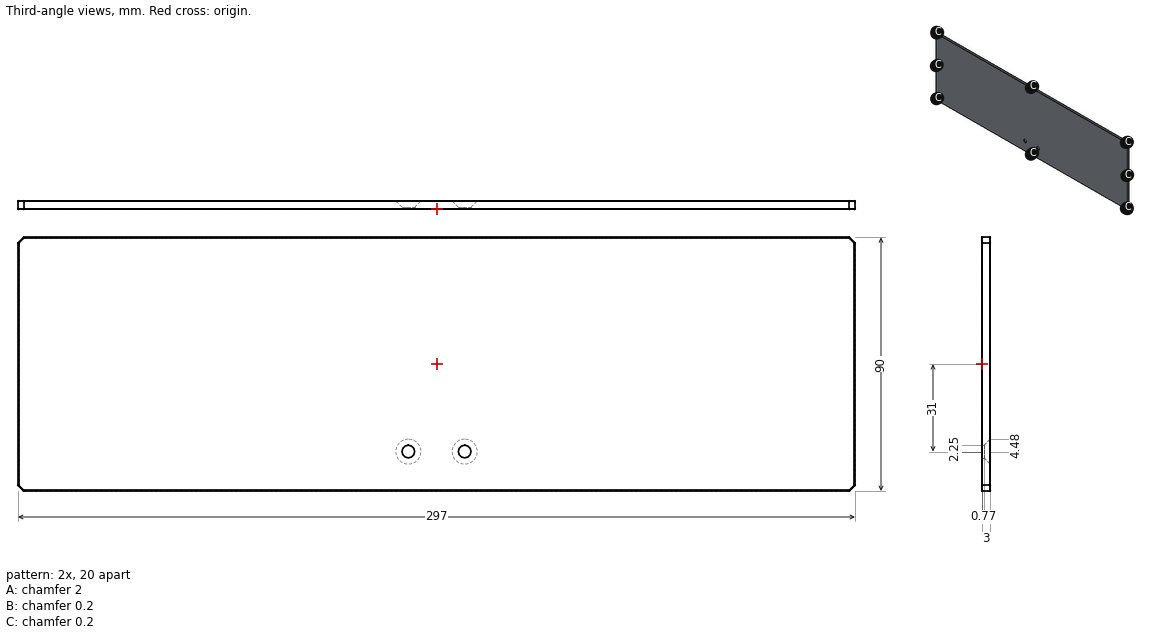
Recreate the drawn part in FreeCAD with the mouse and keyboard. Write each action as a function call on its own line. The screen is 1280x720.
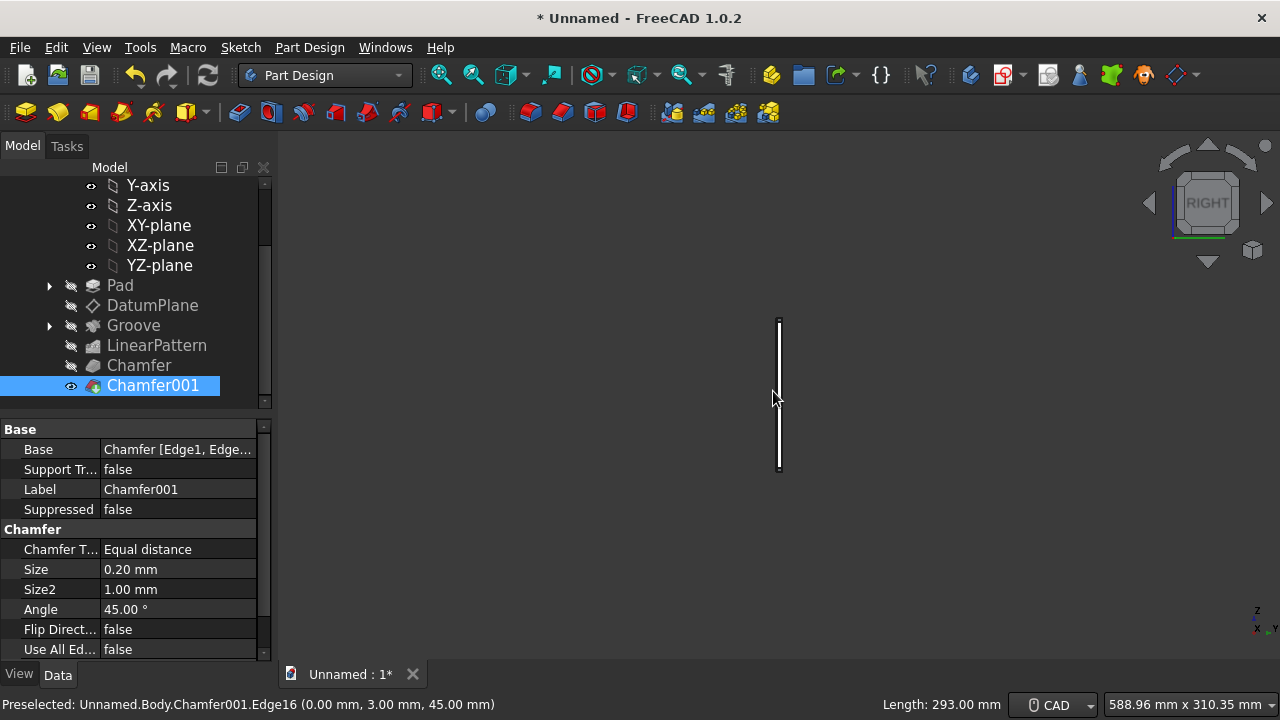
key(v)
key(f)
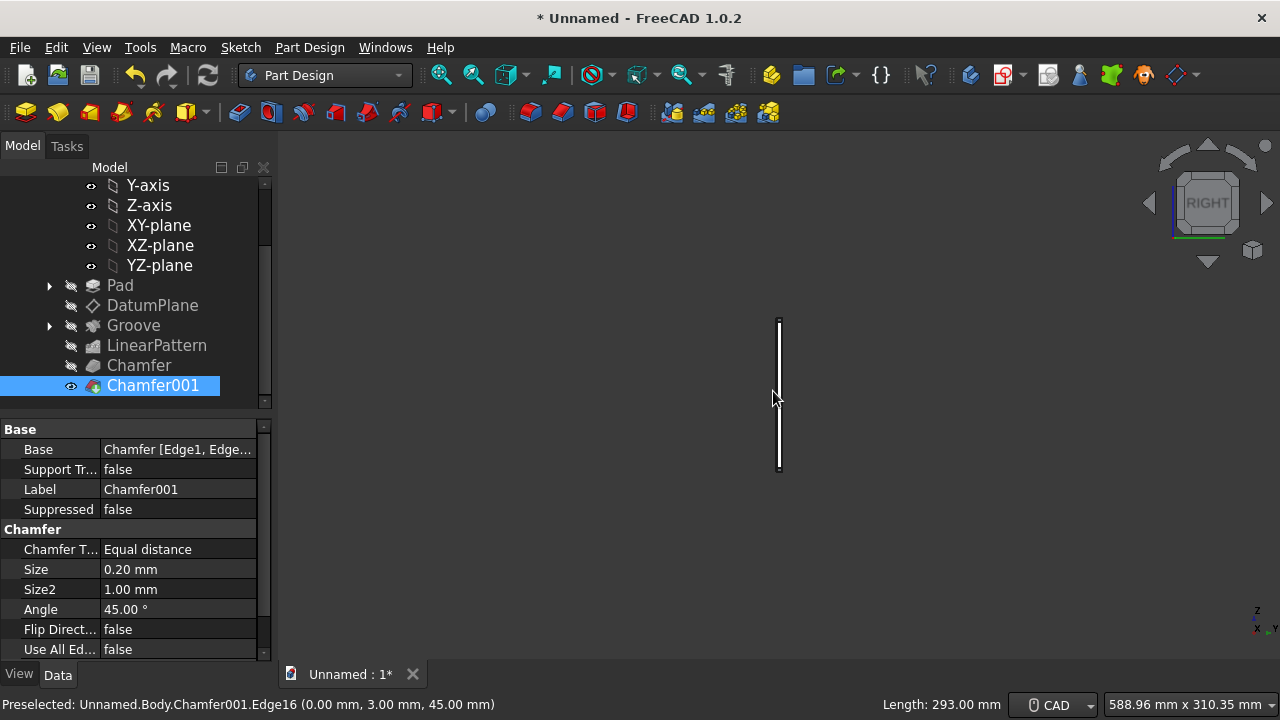
click(782, 394, ctrl)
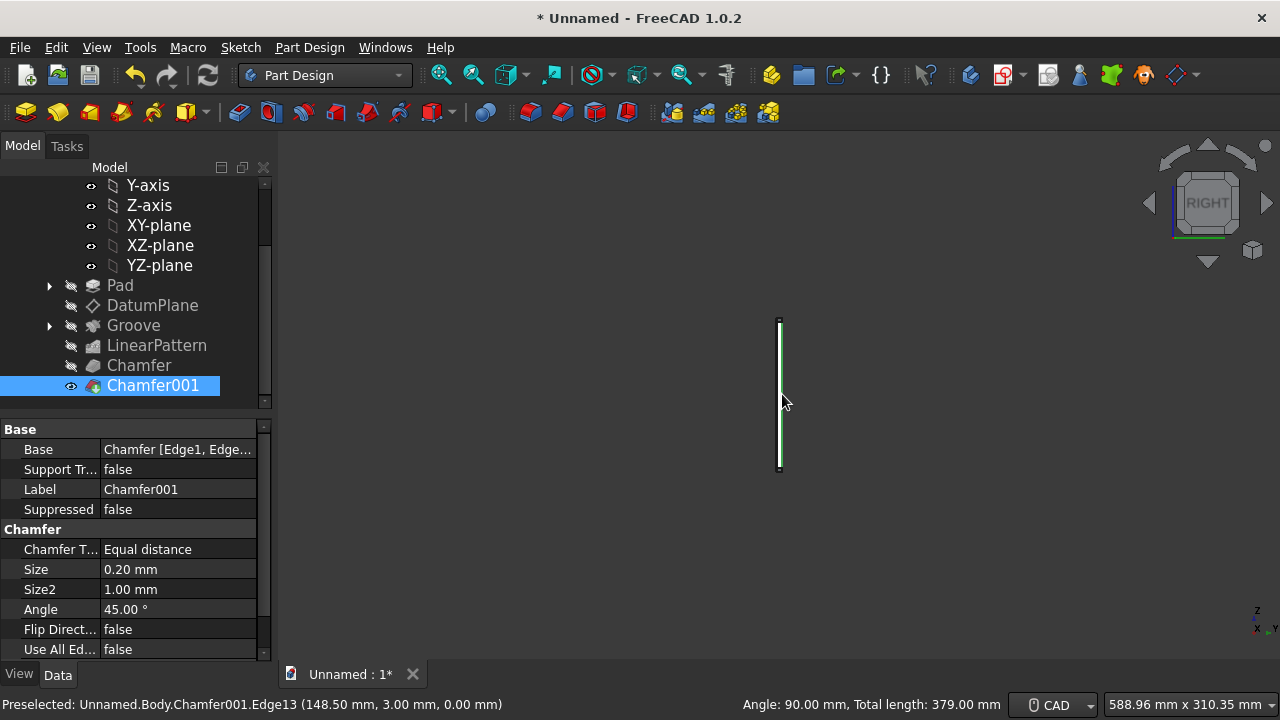
key(5)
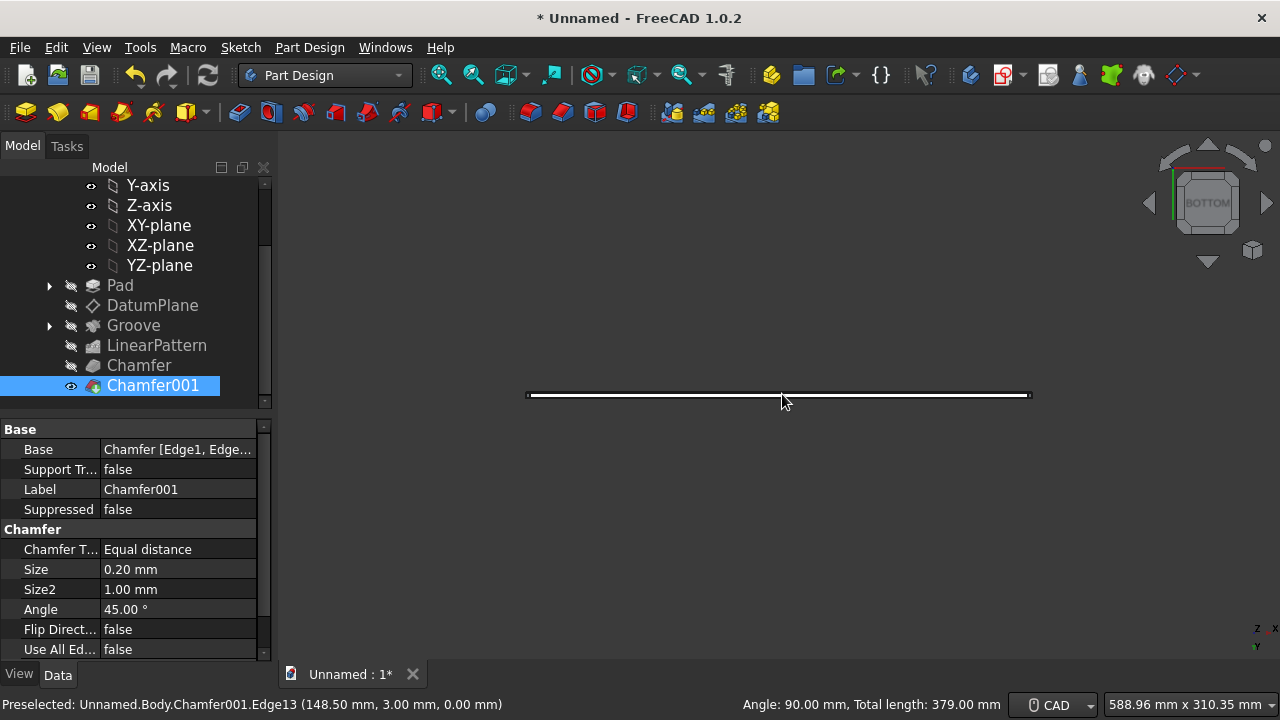
key(4)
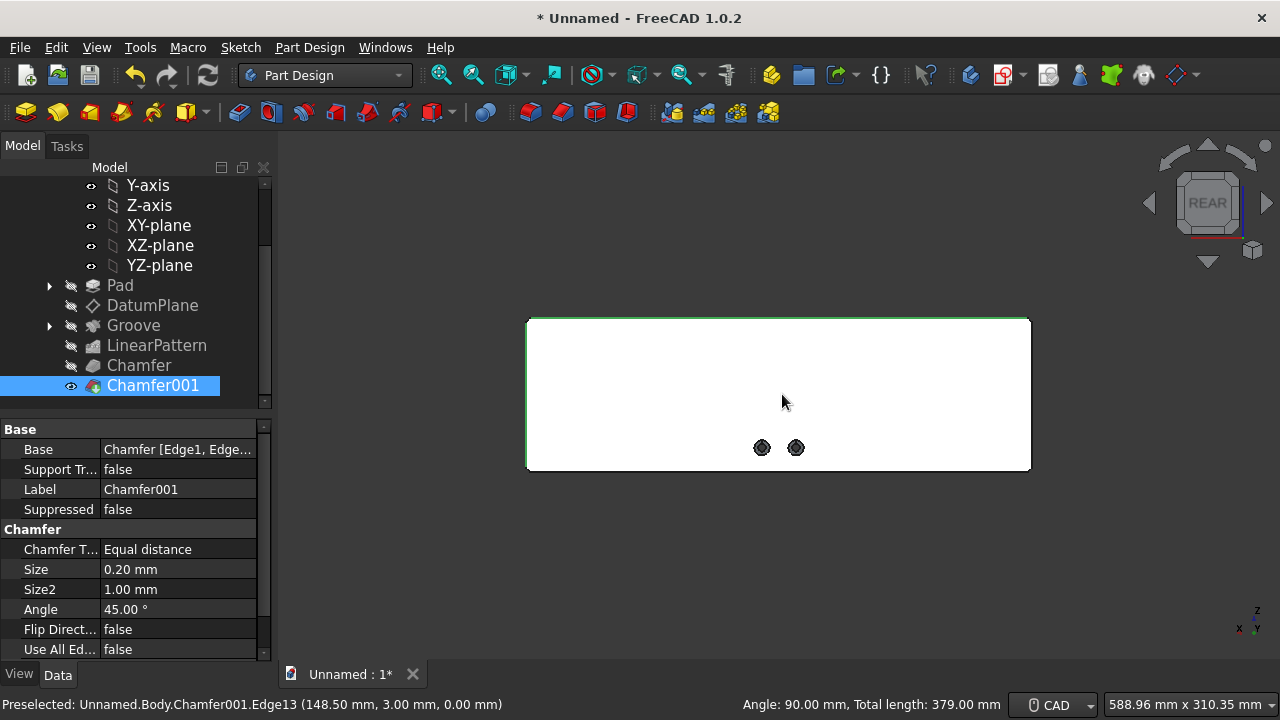
click(779, 471, ctrl)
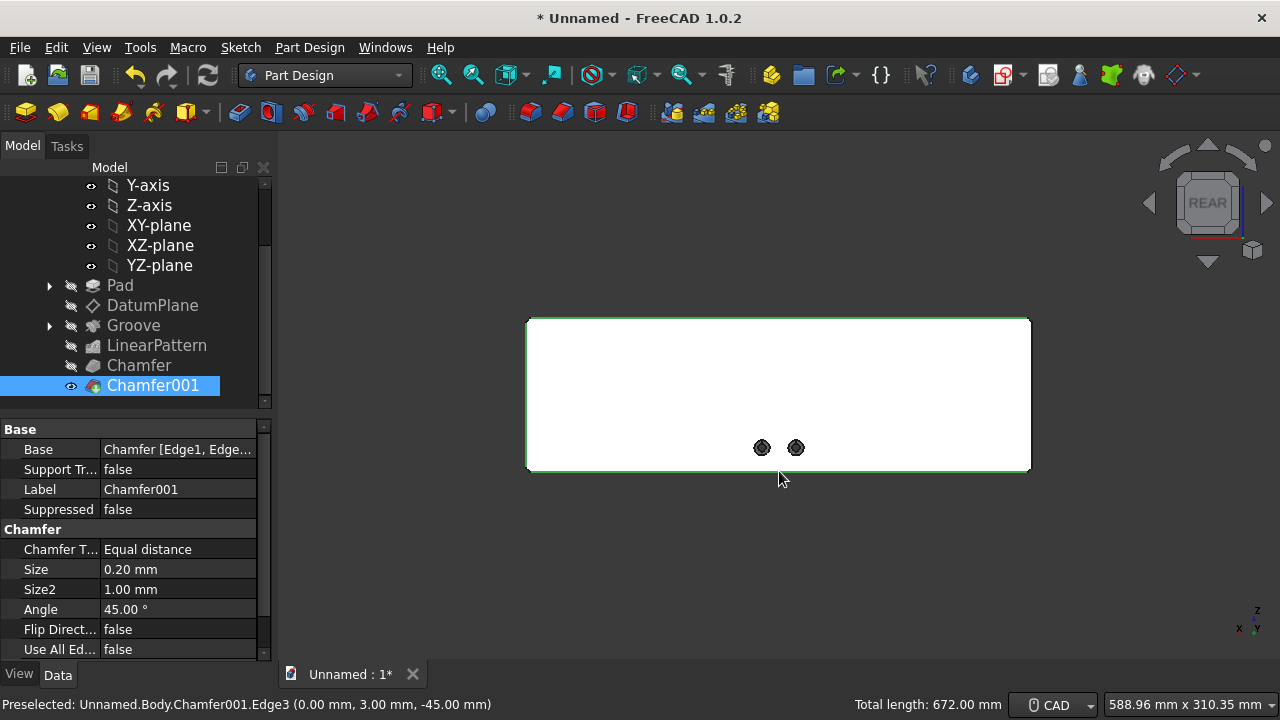
click(1032, 394, ctrl)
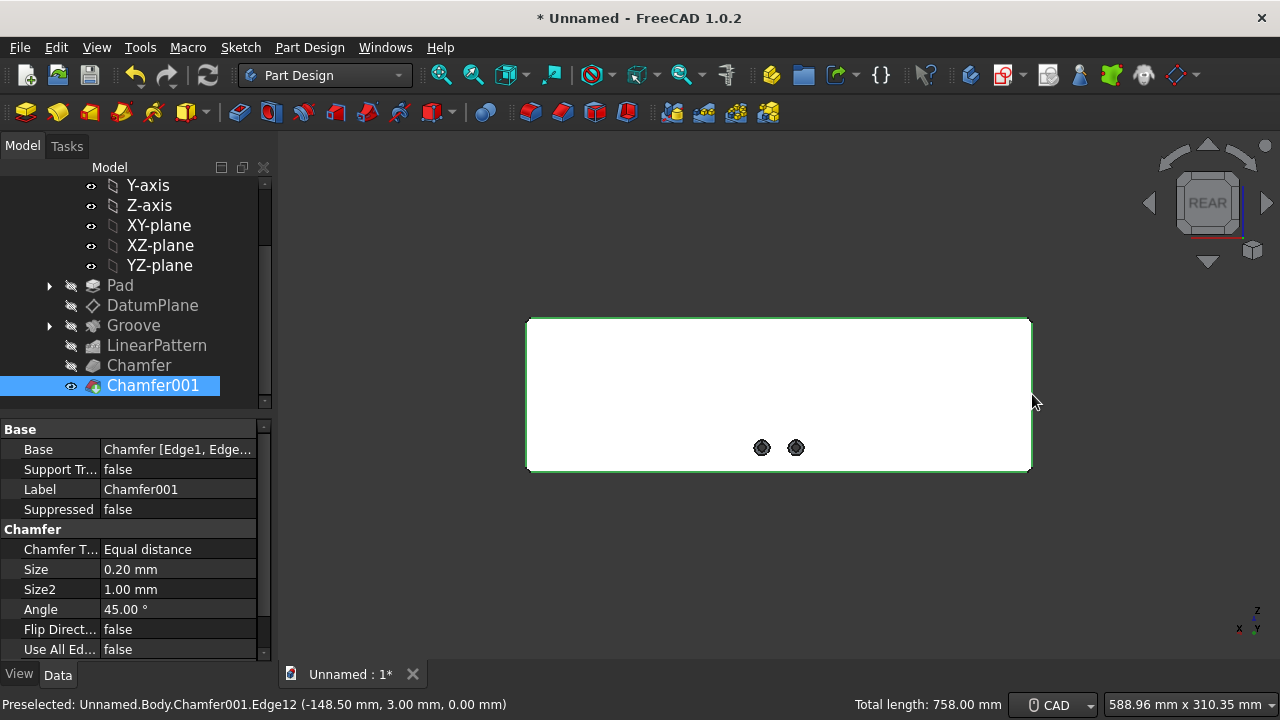
scroll(1030, 469, up, 11)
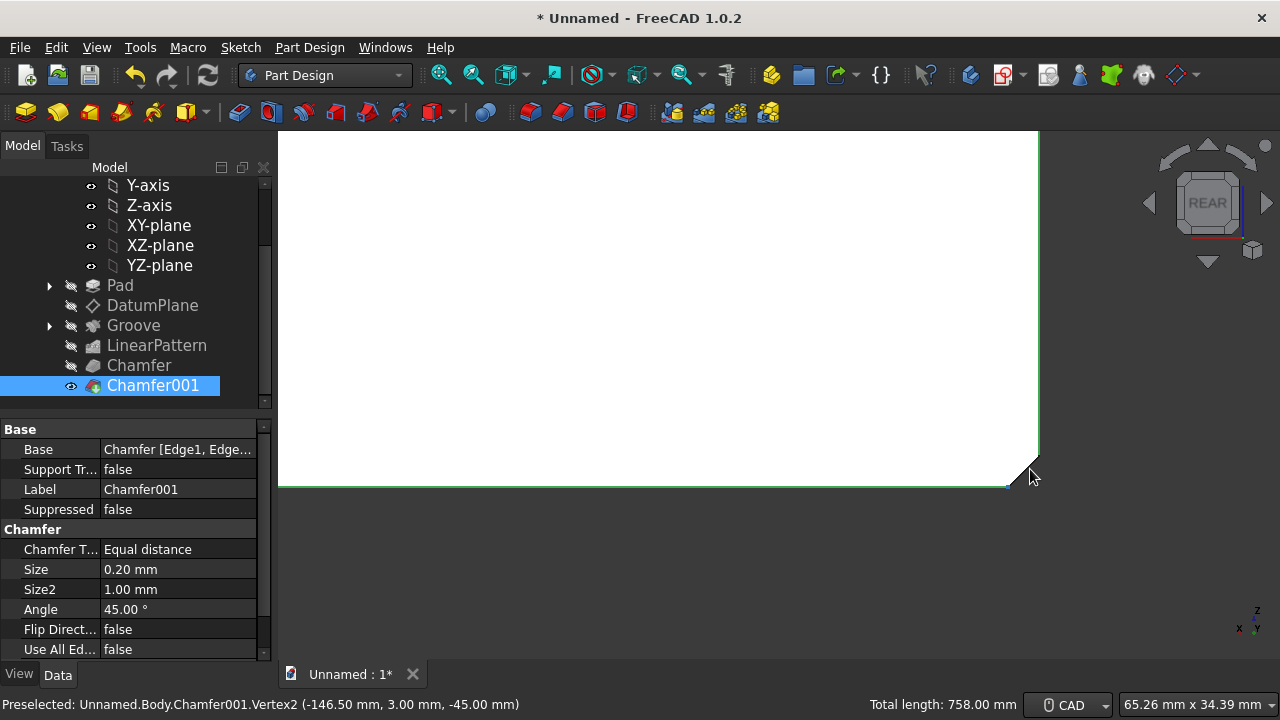
click(1023, 471, ctrl)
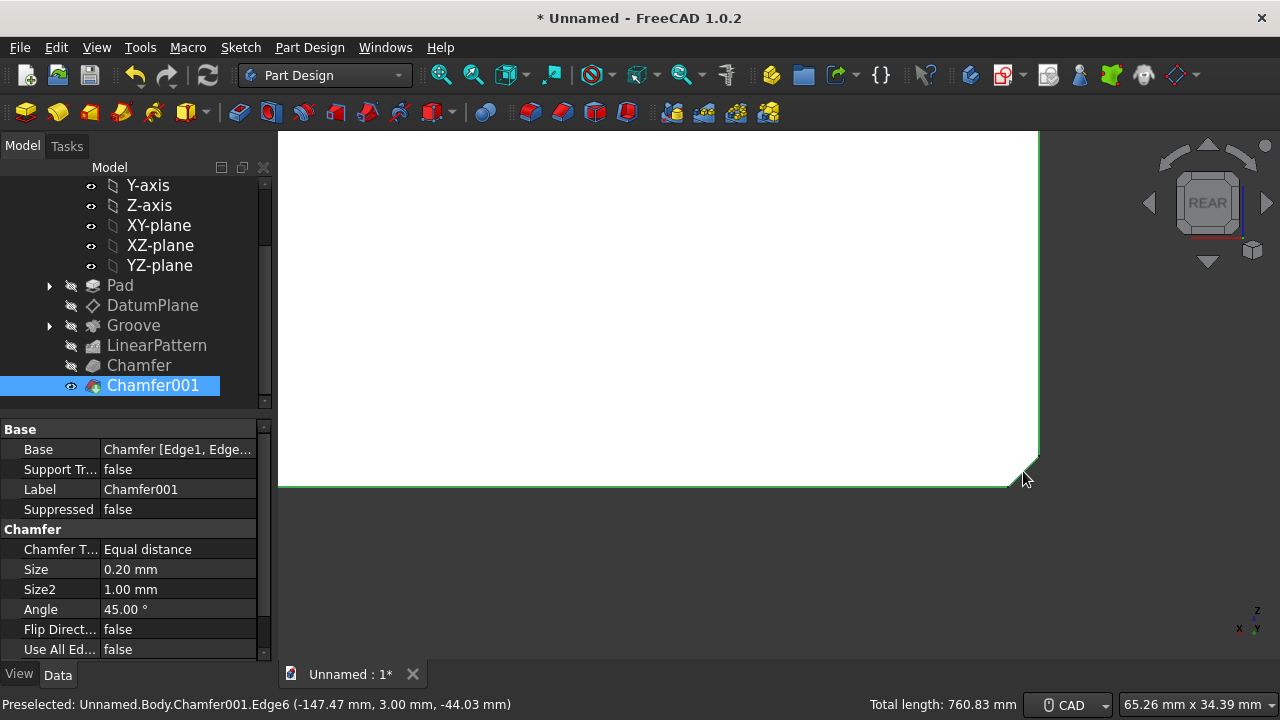
key(v)
key(f)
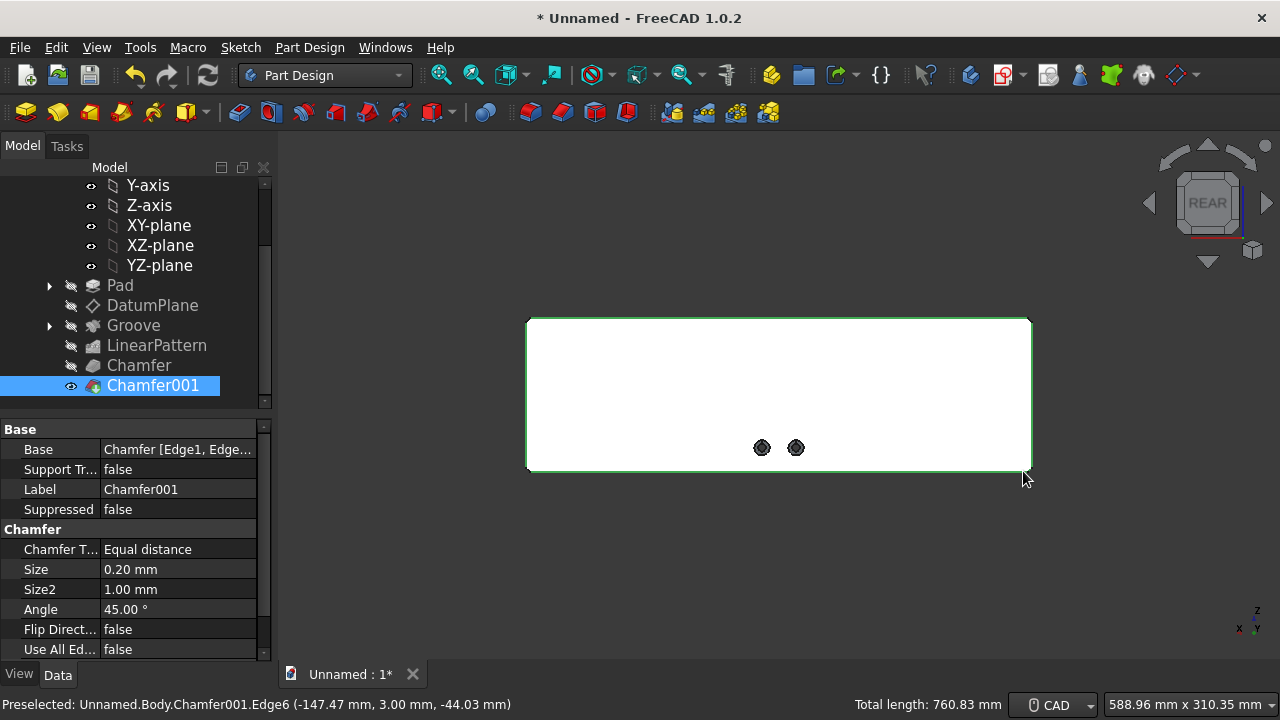
key(6)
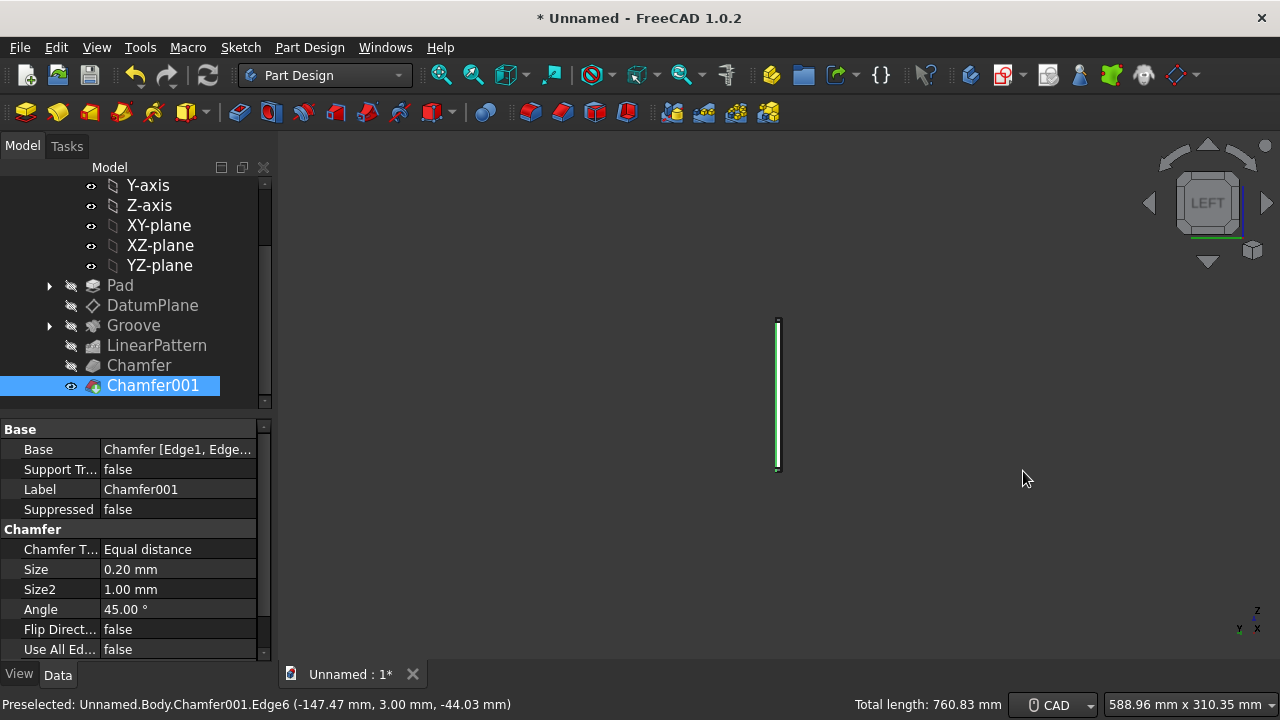
key(v)
key(f)